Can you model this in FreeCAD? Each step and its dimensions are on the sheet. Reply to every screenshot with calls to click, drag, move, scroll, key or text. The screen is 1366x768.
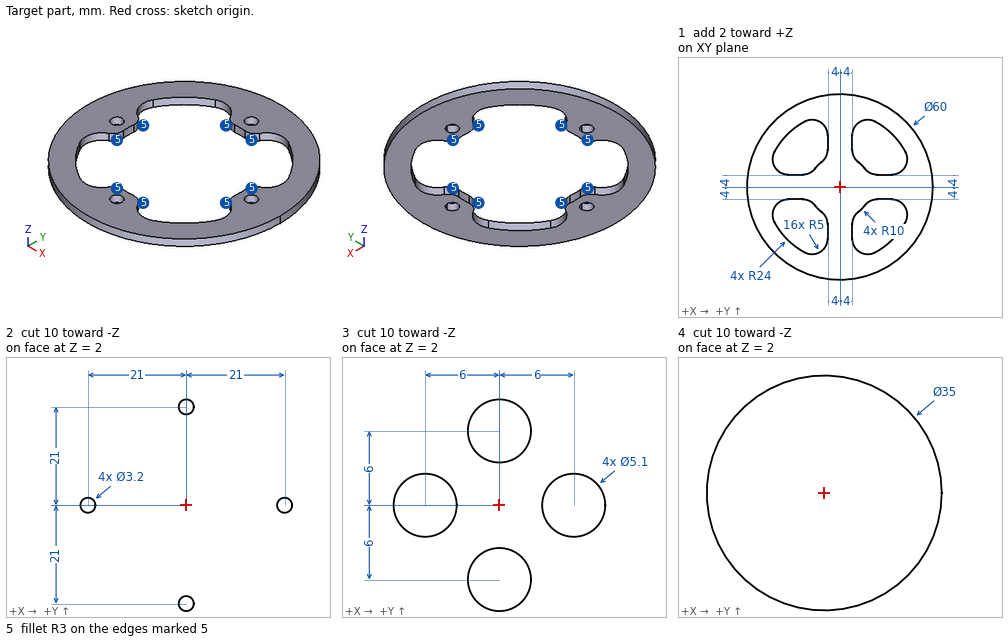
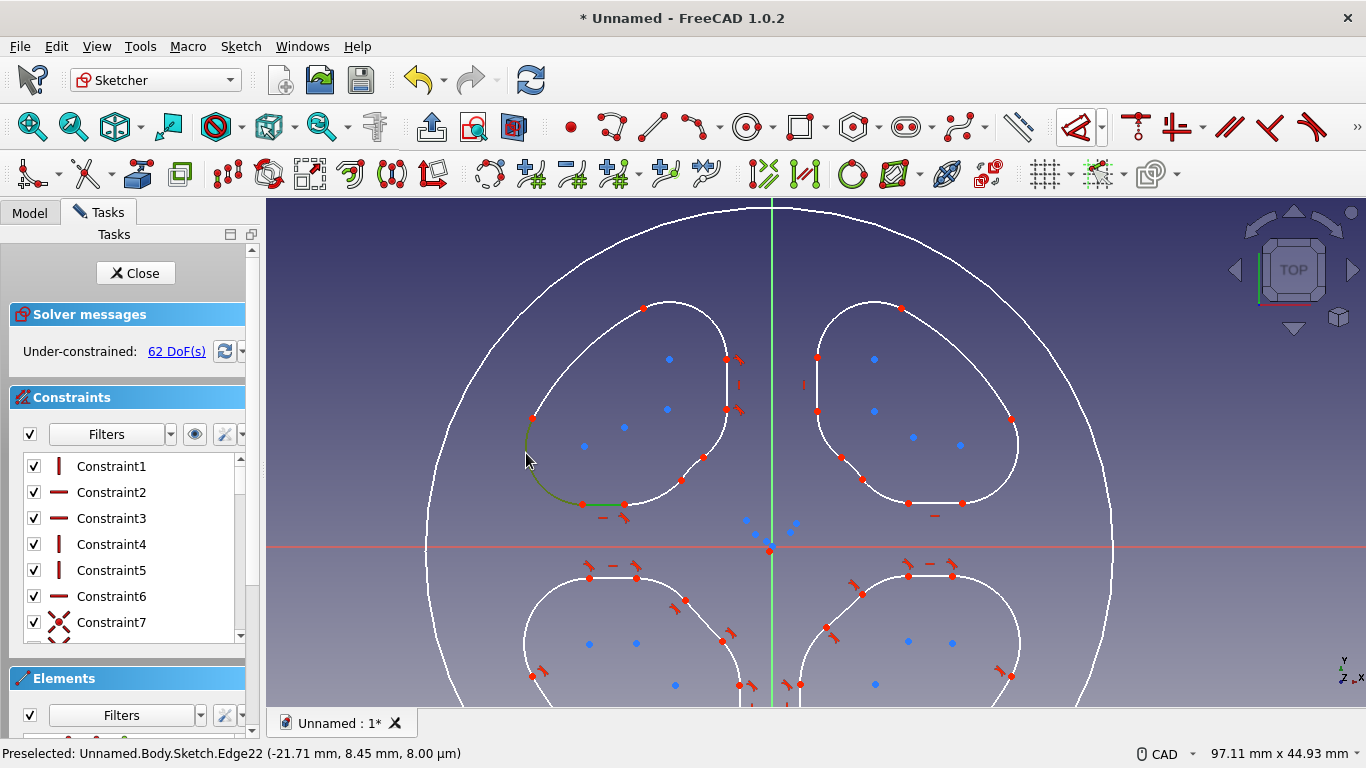
key(t)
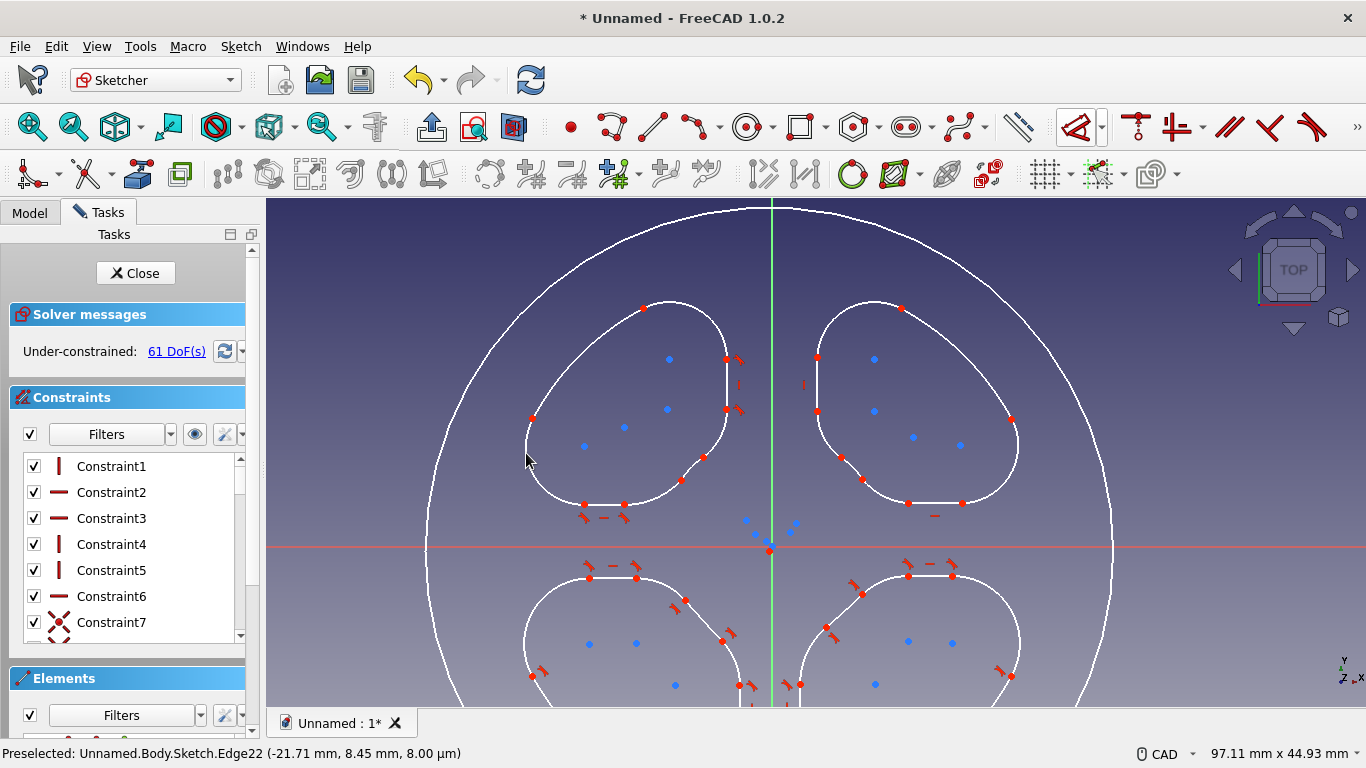
click(715, 445)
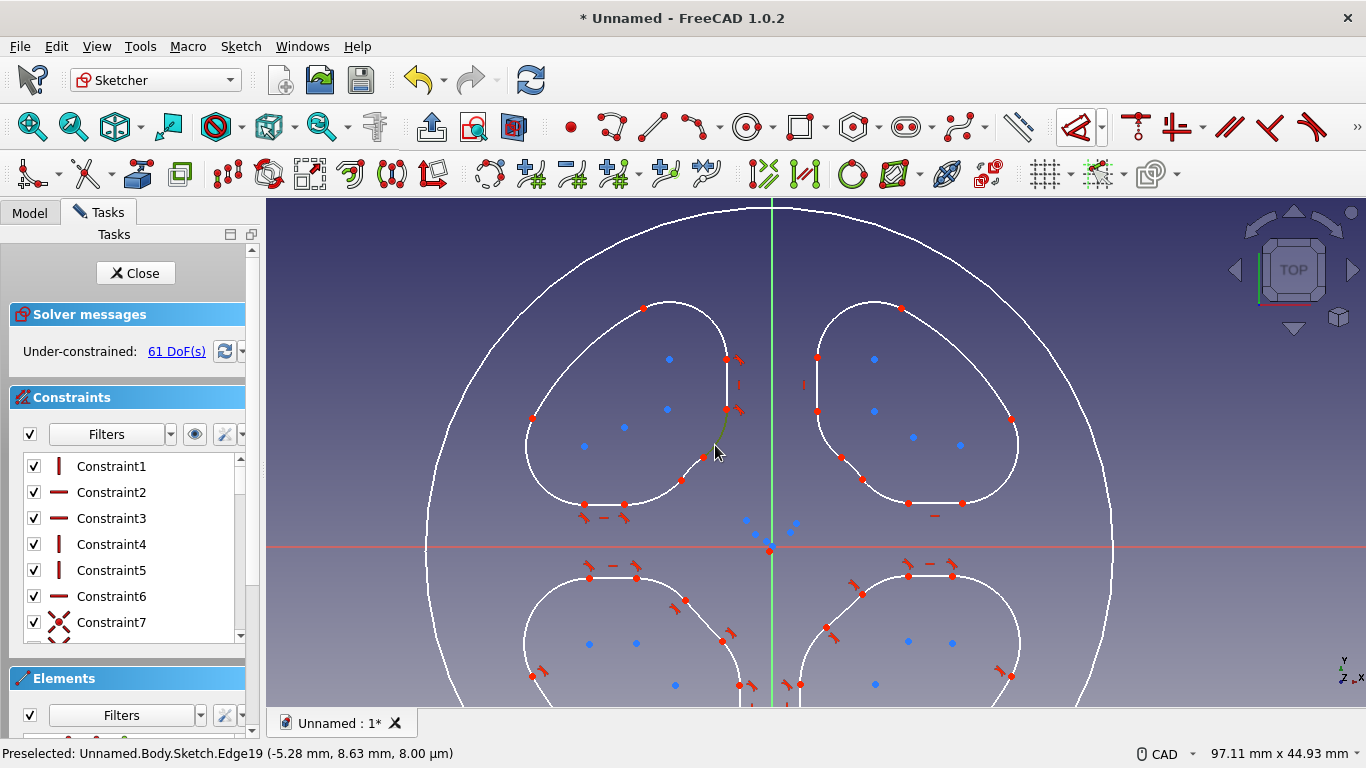
scroll(696, 463, up, 2)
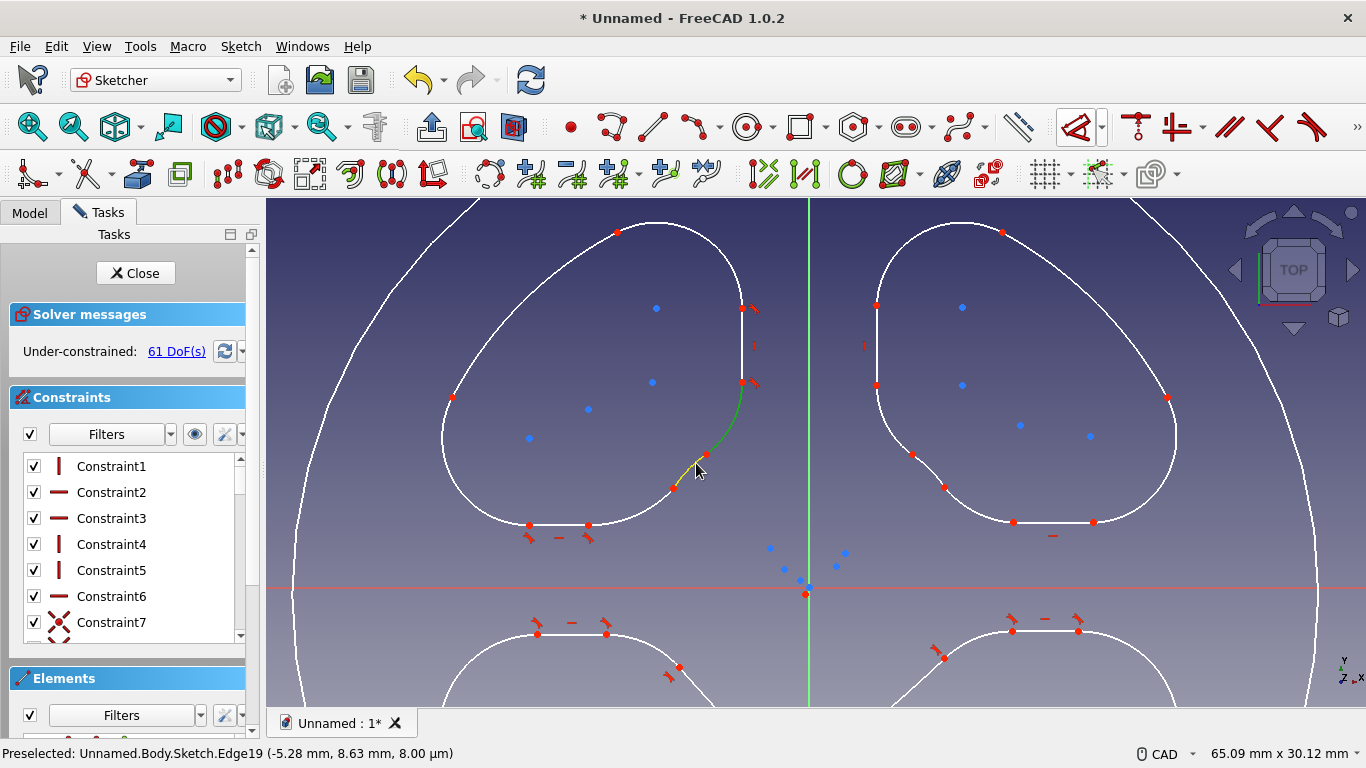
click(695, 463)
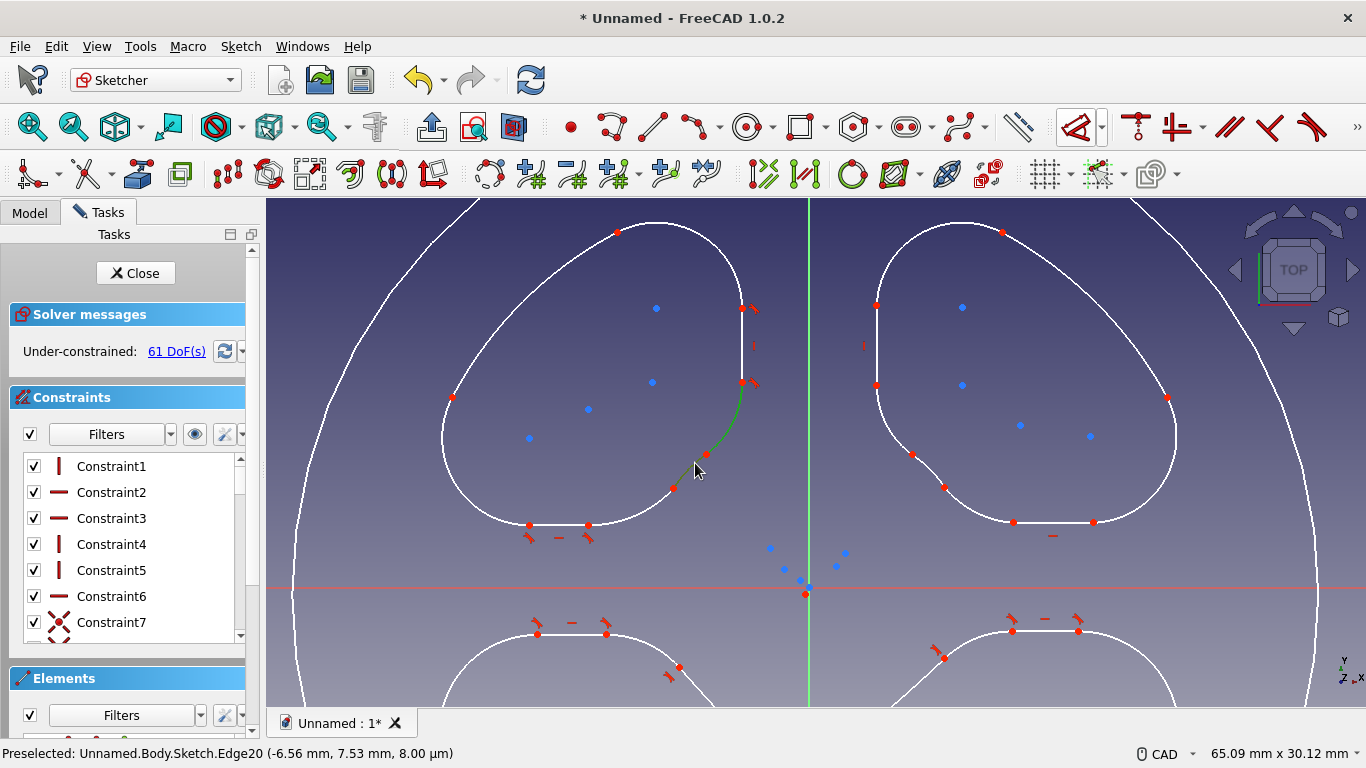
key(t)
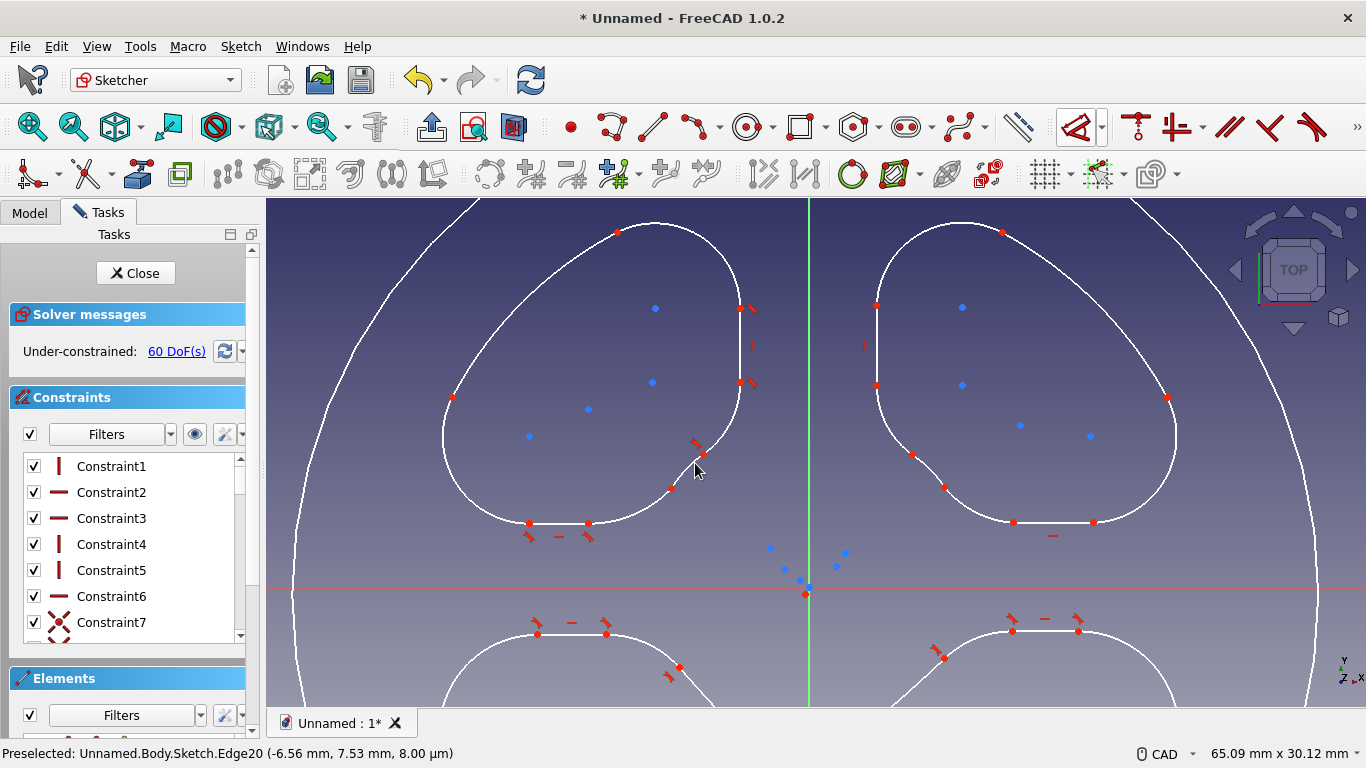
click(692, 463)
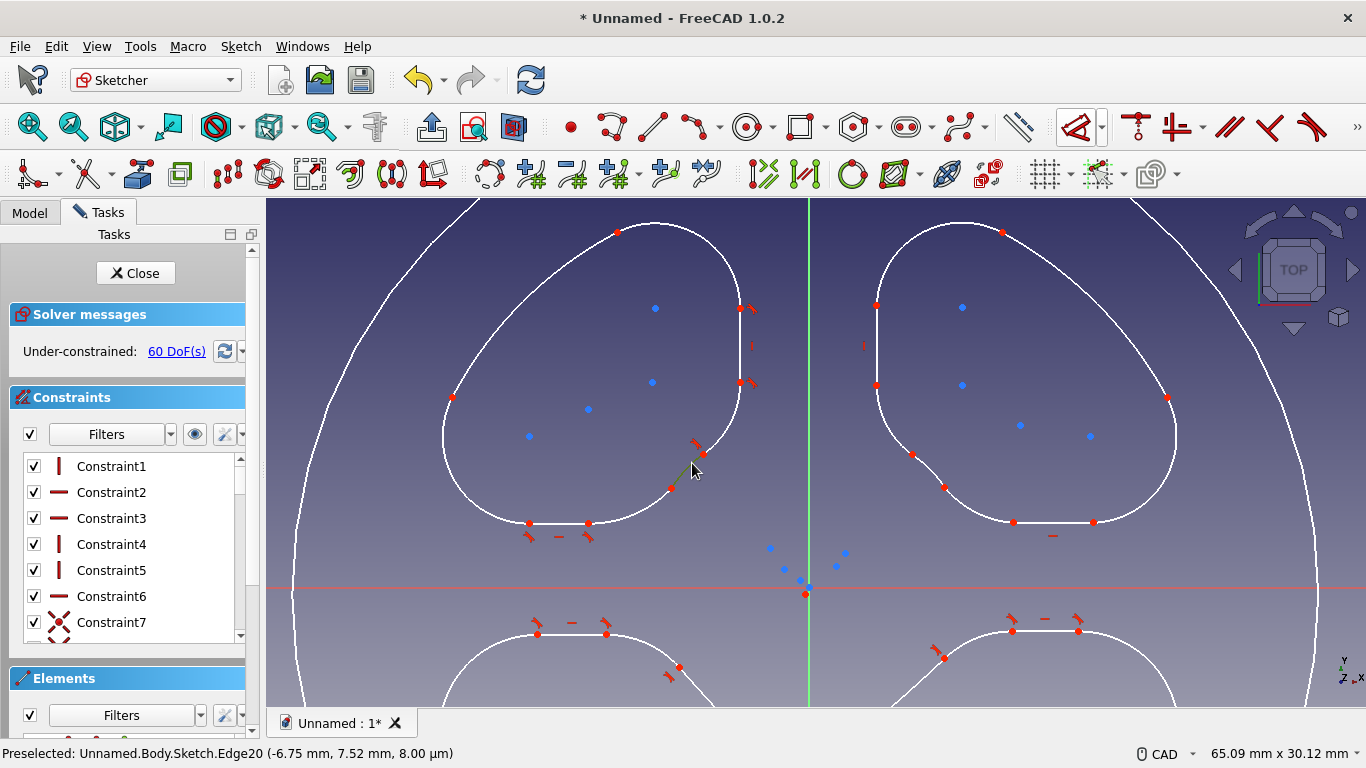
click(616, 520)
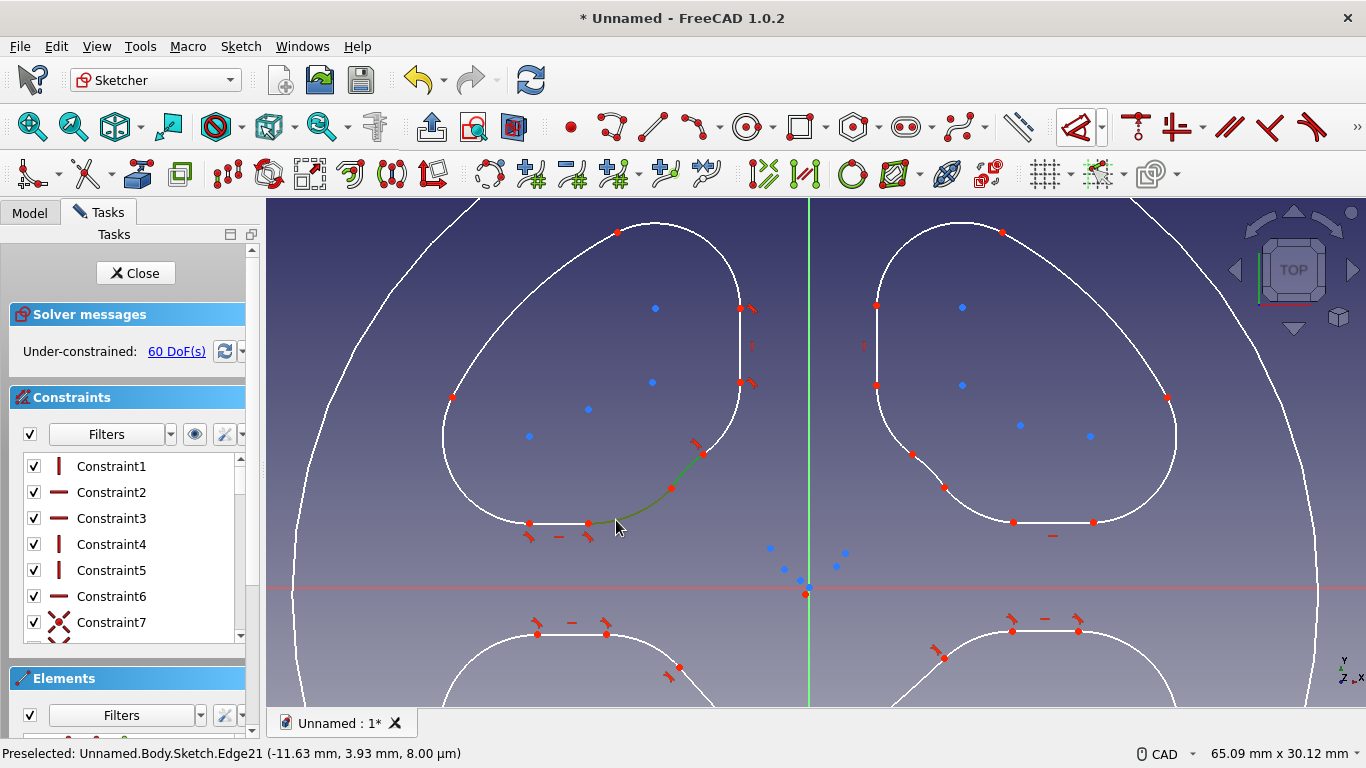
click(1312, 128)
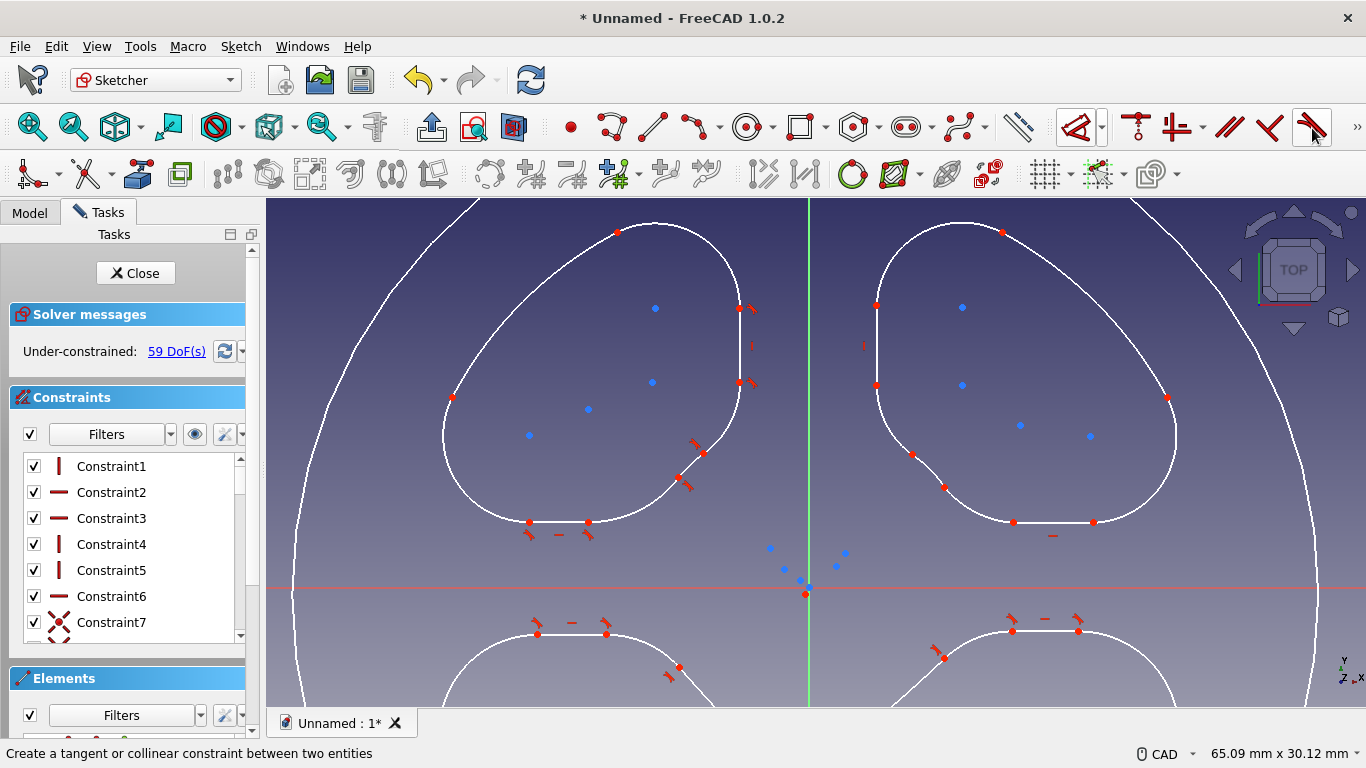
click(444, 448)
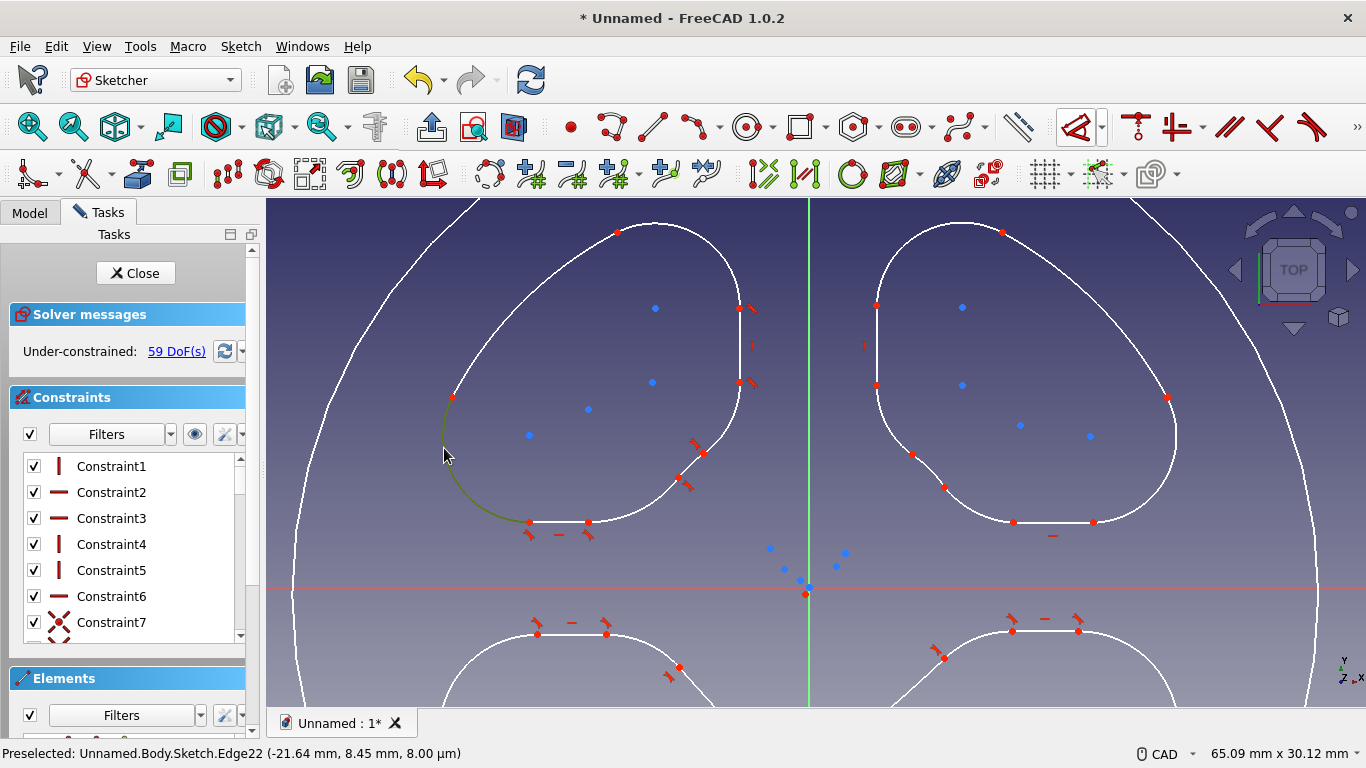
click(558, 271)